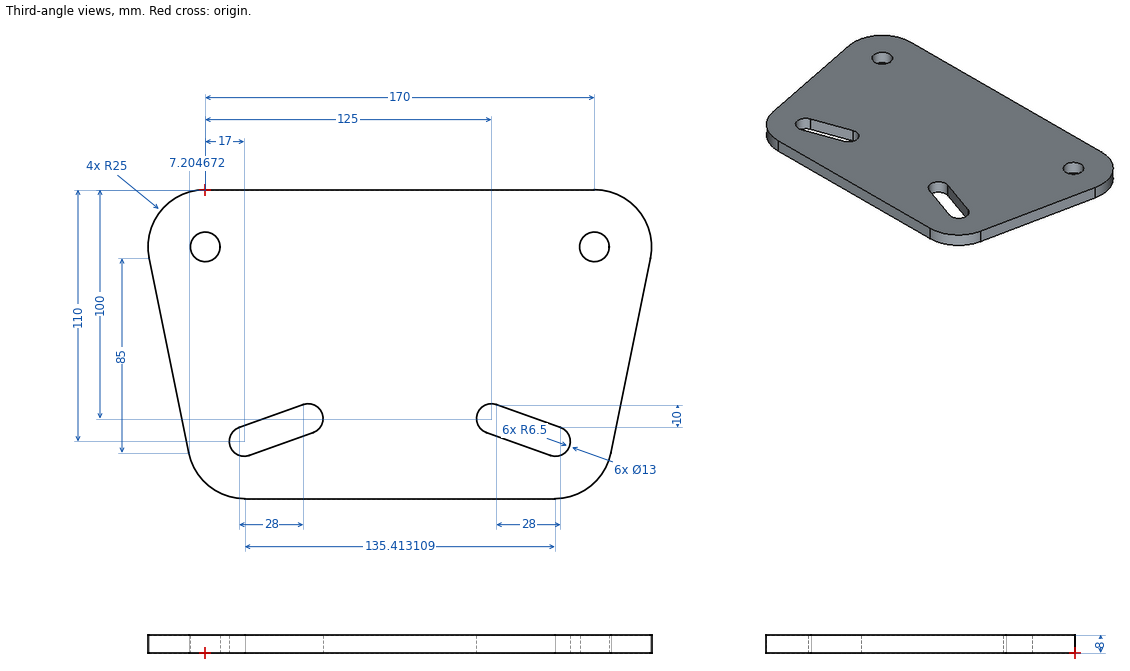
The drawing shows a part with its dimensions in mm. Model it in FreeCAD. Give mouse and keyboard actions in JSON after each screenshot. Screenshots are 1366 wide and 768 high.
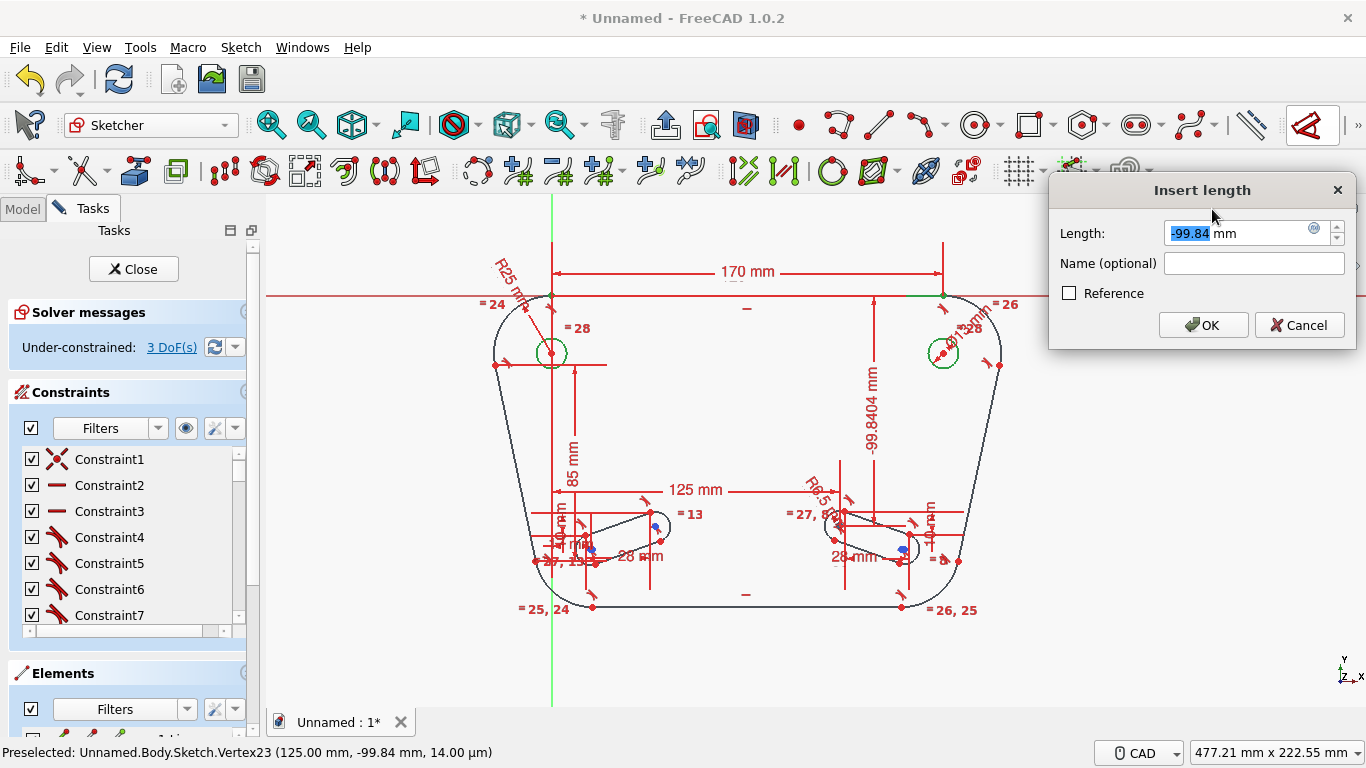
{"action": "type", "text": "-100"}
{"action": "key", "text": "Return"}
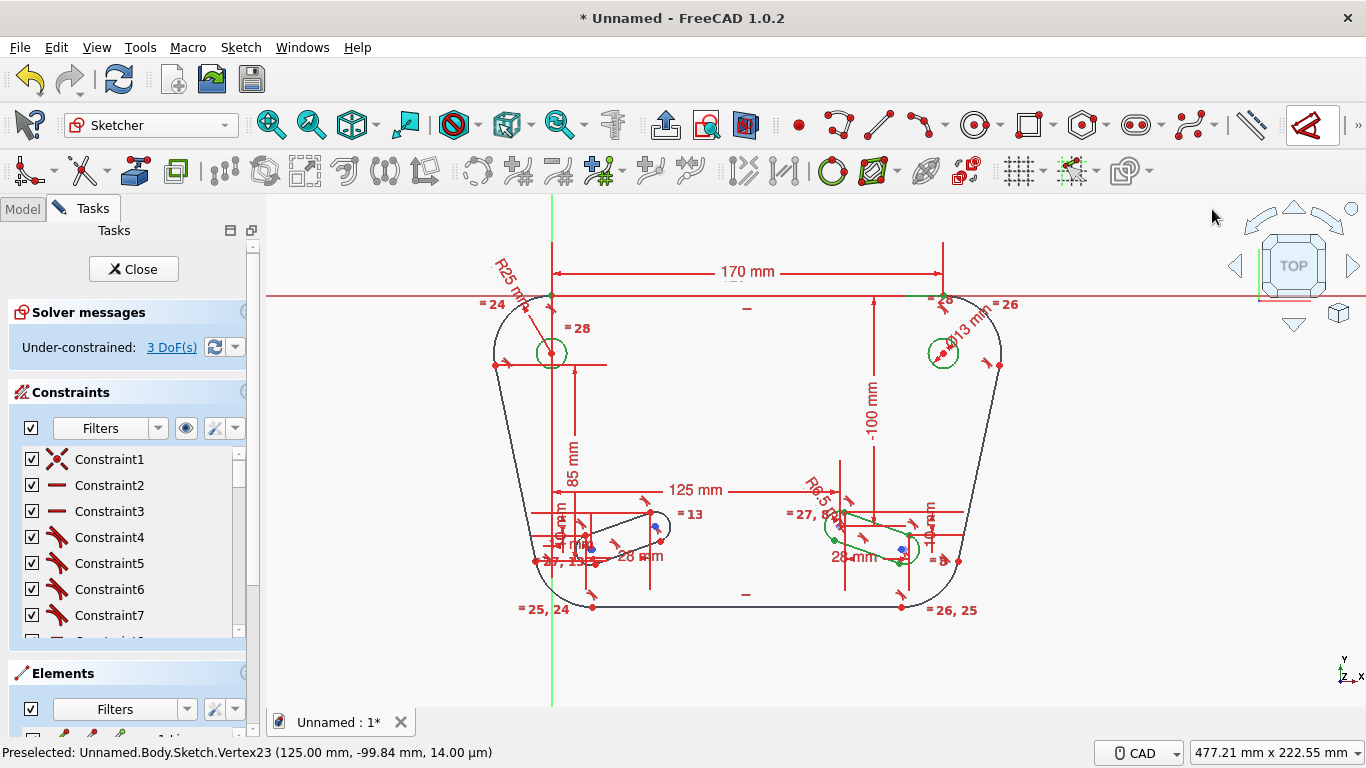
{"action": "scroll", "coordinate": [591, 550], "scroll_direction": "up", "scroll_amount": 11}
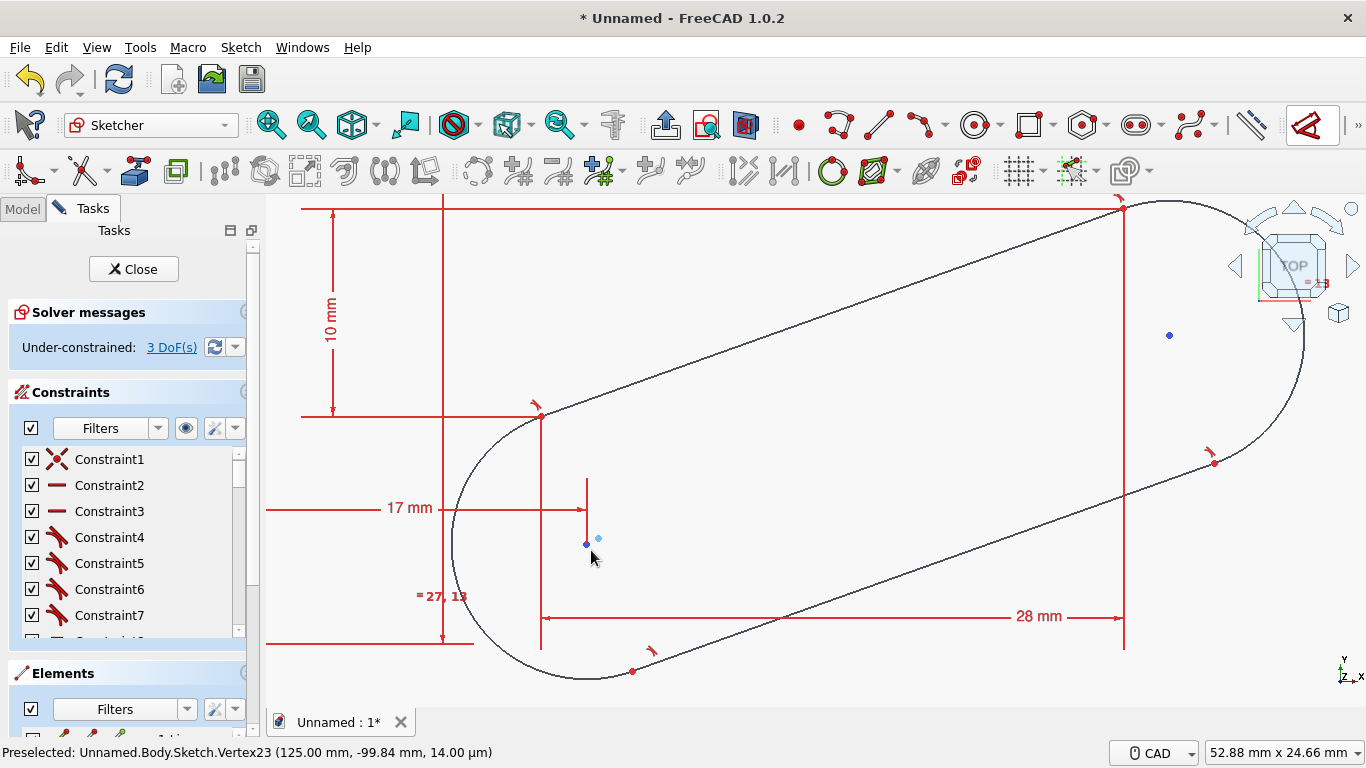
{"action": "left_click", "coordinate": [587, 544]}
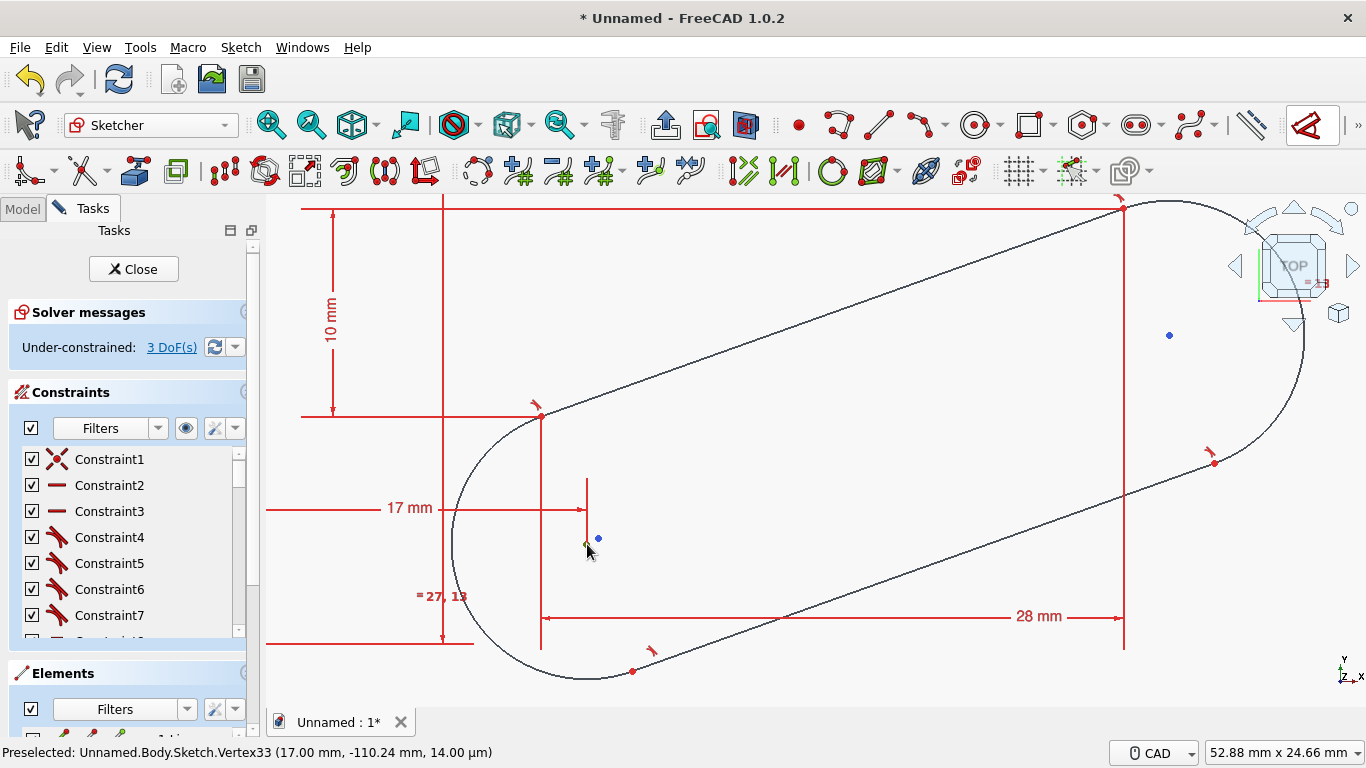
{"action": "left_click", "coordinate": [1334, 126]}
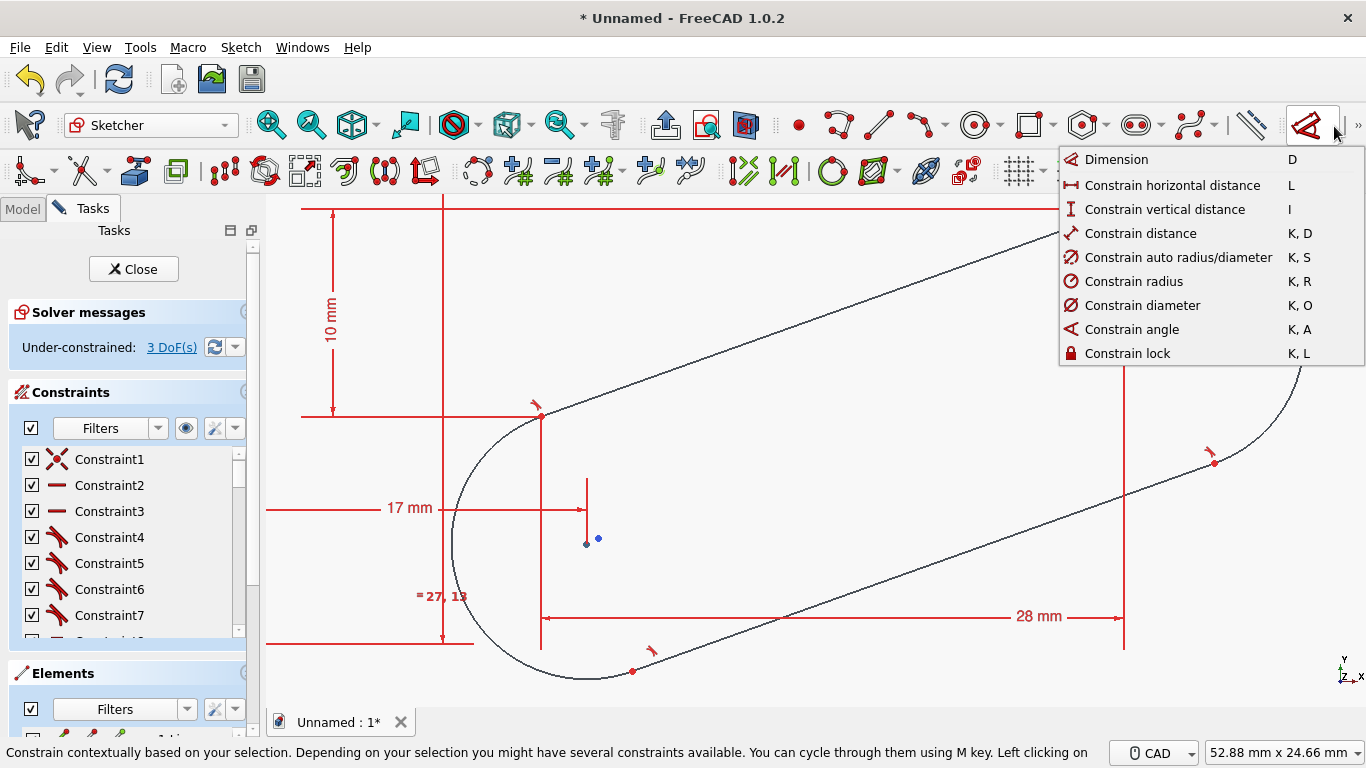
{"action": "left_click", "coordinate": [1212, 209]}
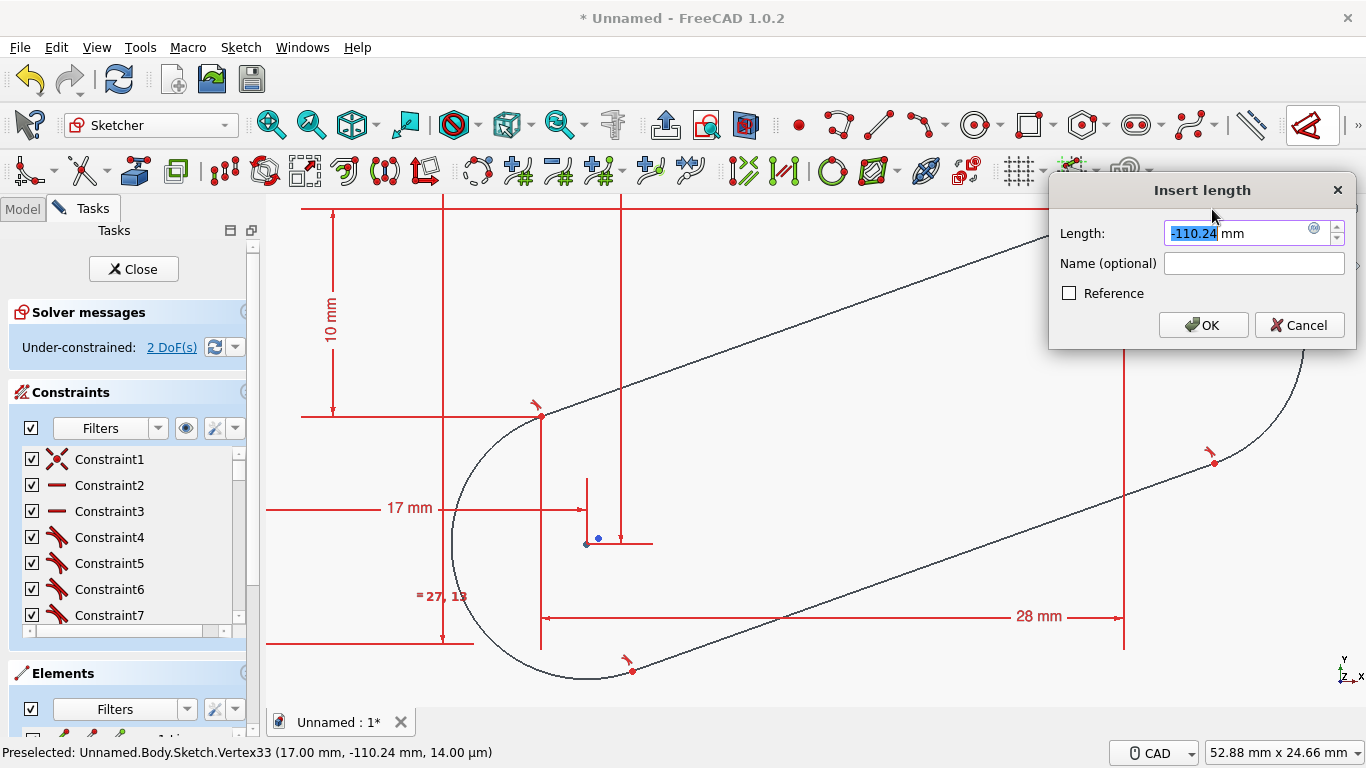
{"action": "type", "text": "-110"}
{"action": "key", "text": "Return"}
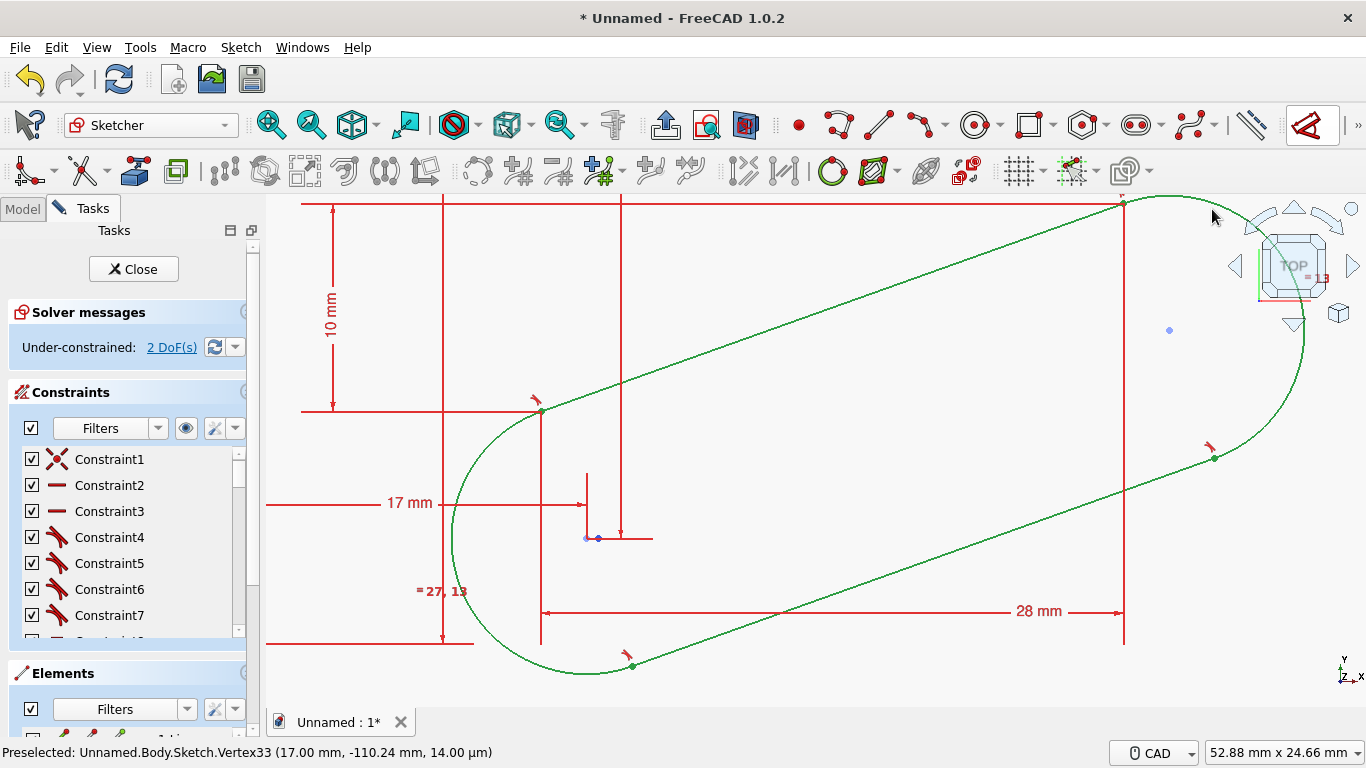
{"action": "scroll", "coordinate": [591, 550], "scroll_direction": "down", "scroll_amount": 11}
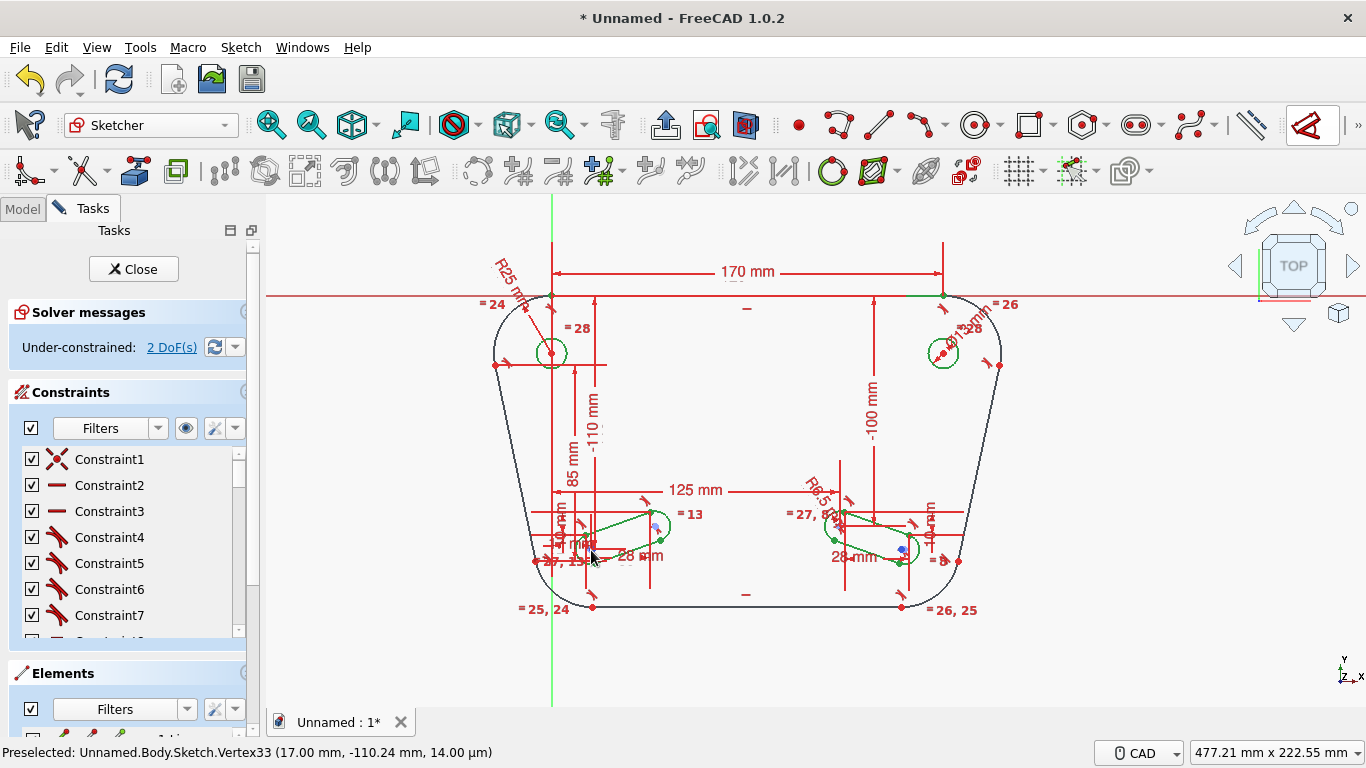
{"action": "scroll", "coordinate": [536, 561], "scroll_direction": "up", "scroll_amount": 5}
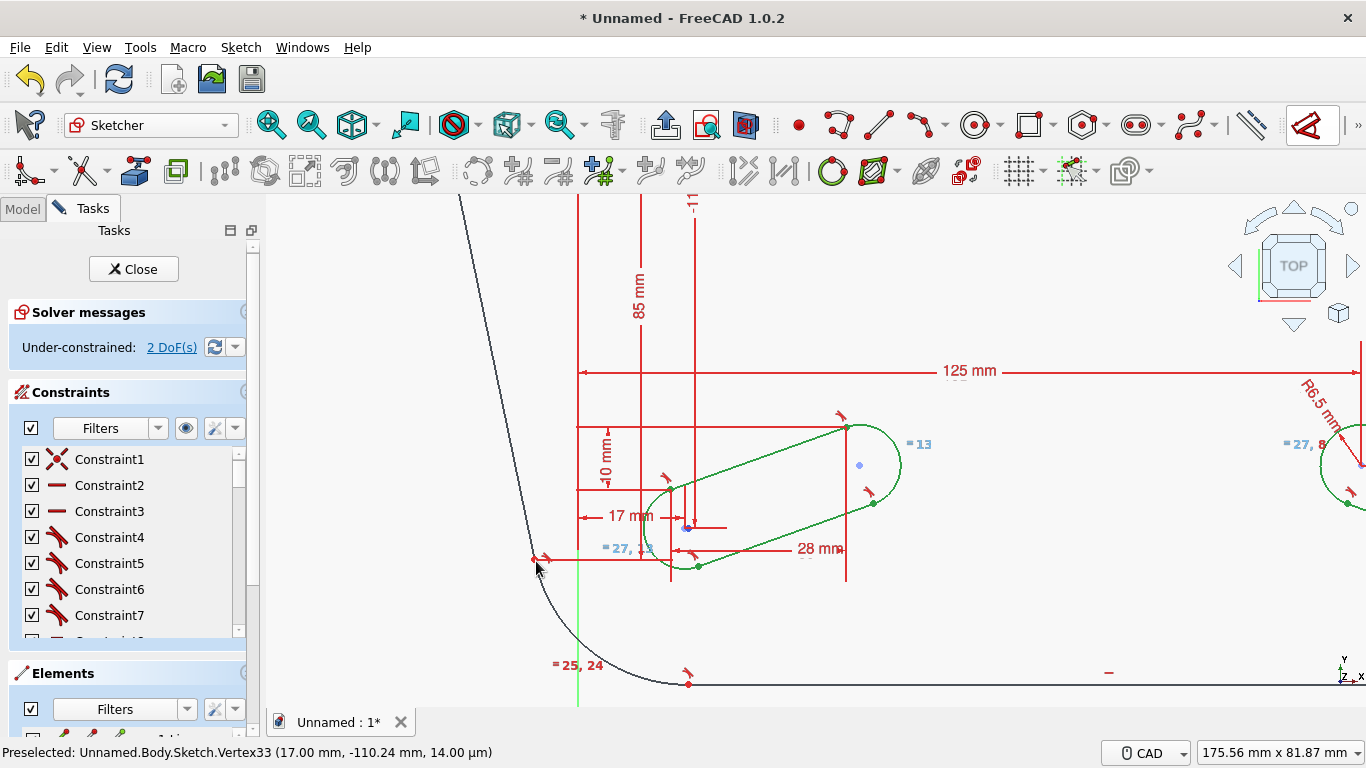
{"action": "left_click", "coordinate": [535, 560]}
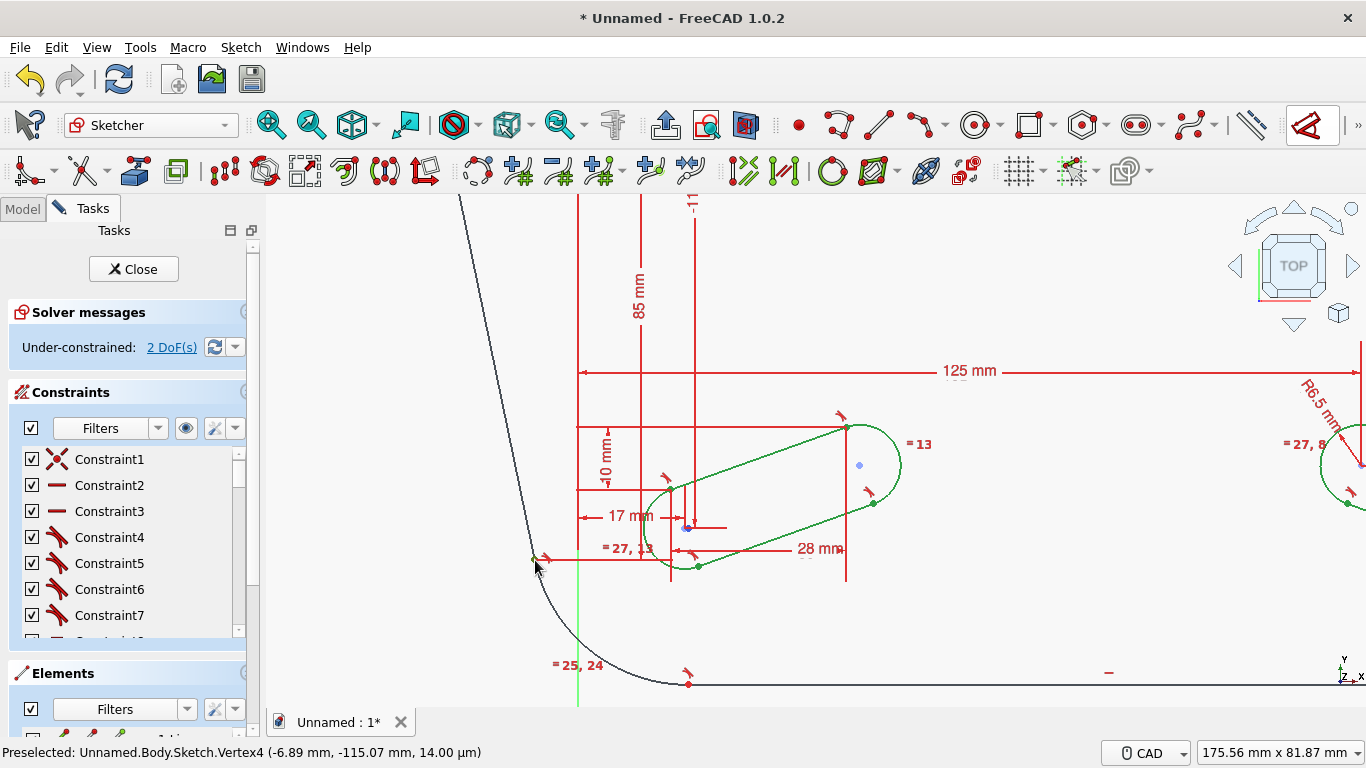
{"action": "left_click", "coordinate": [1334, 126]}